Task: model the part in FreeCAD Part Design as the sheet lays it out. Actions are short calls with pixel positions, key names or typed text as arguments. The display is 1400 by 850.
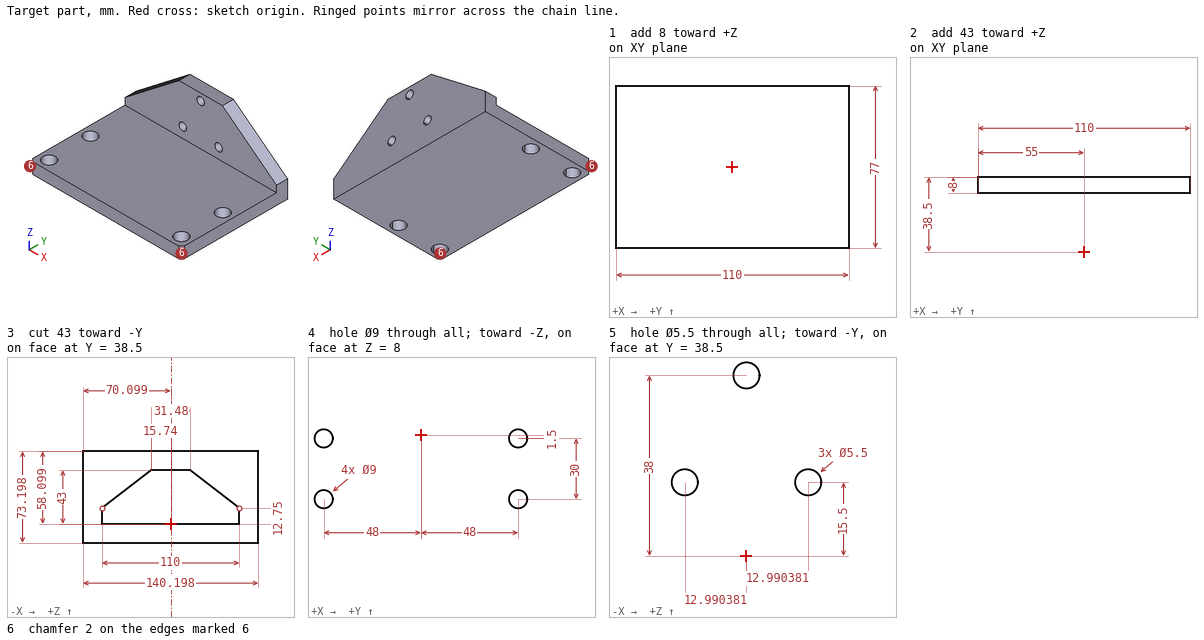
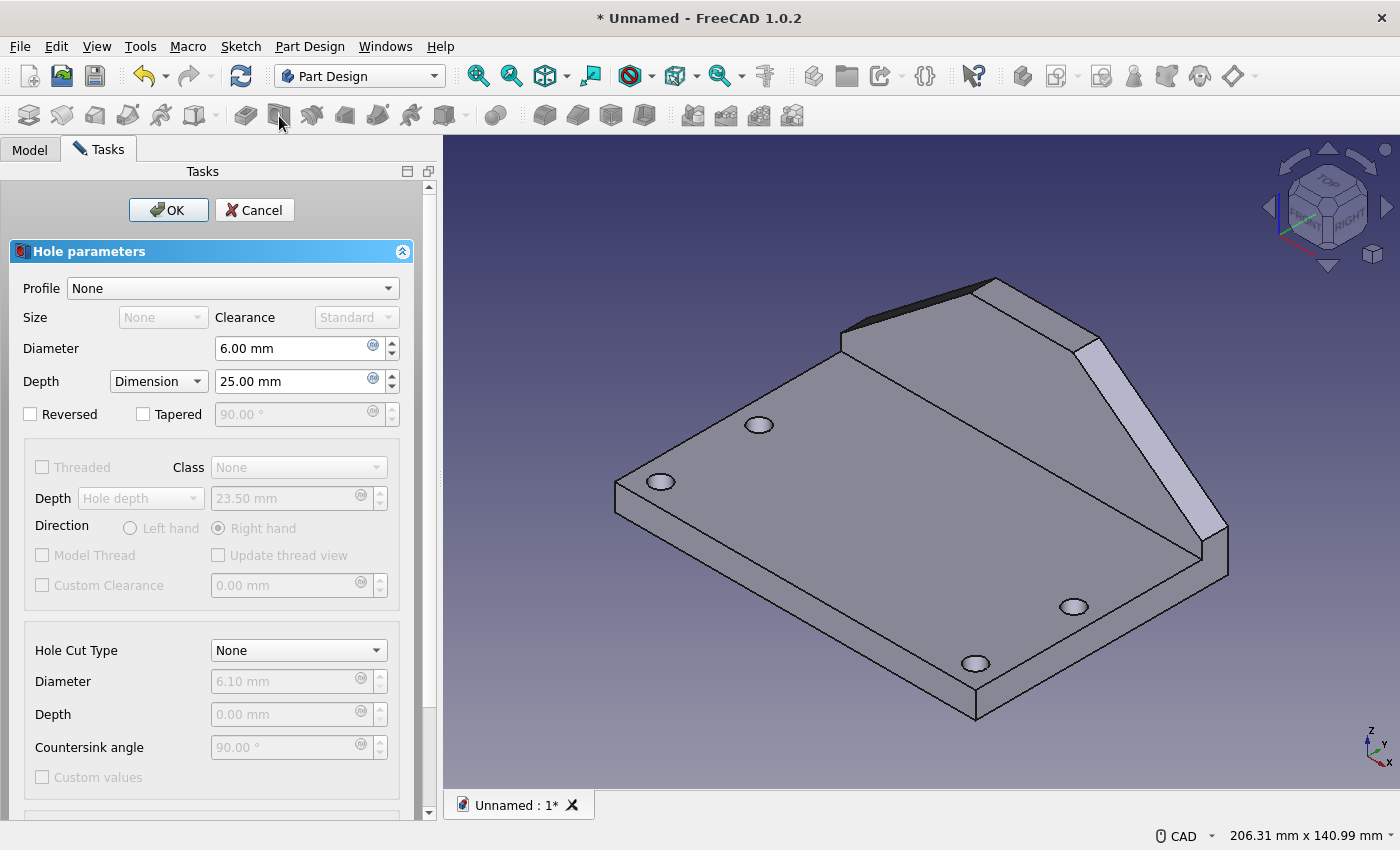
triple_click(300, 348)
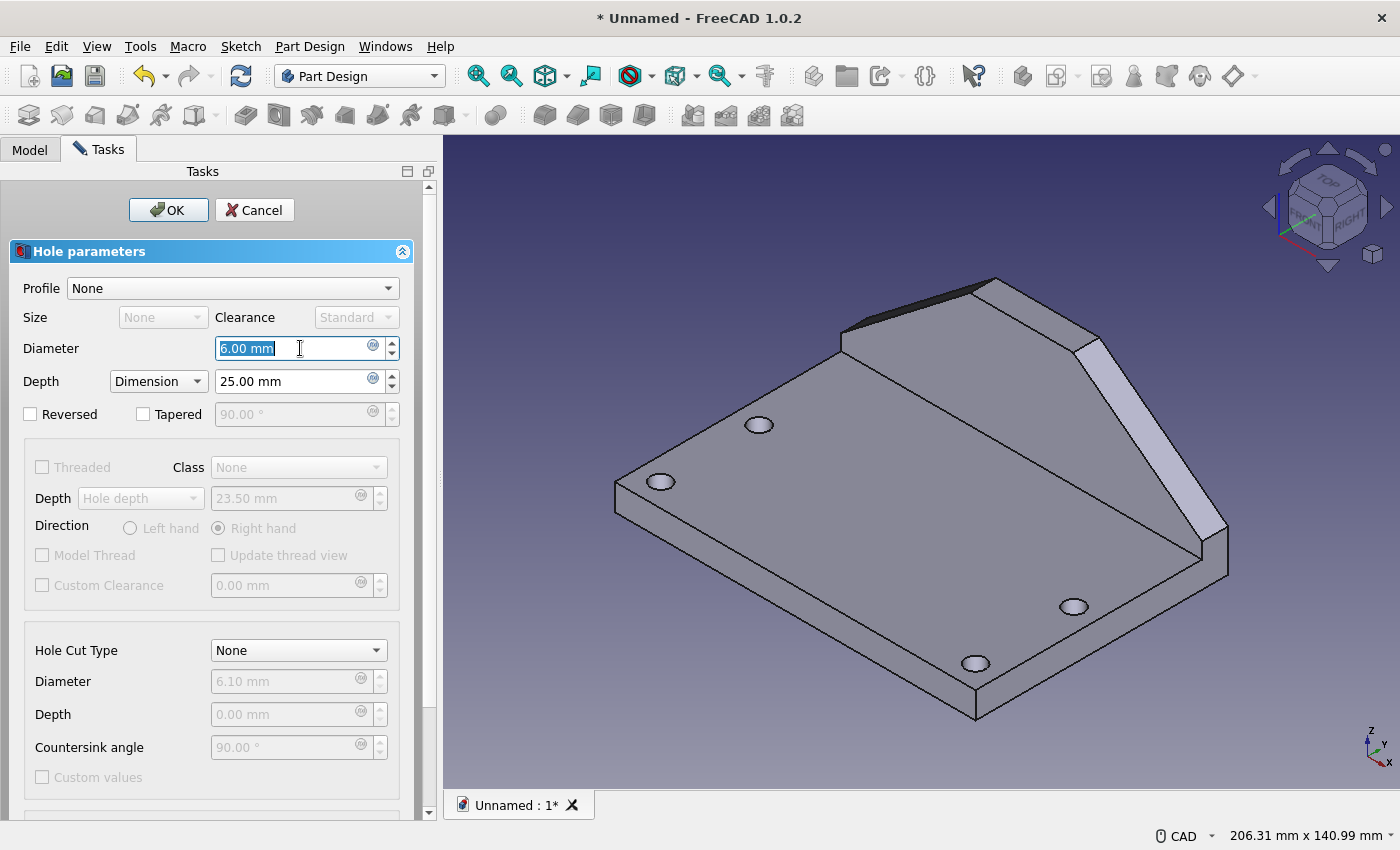
text(9)
key(Tab)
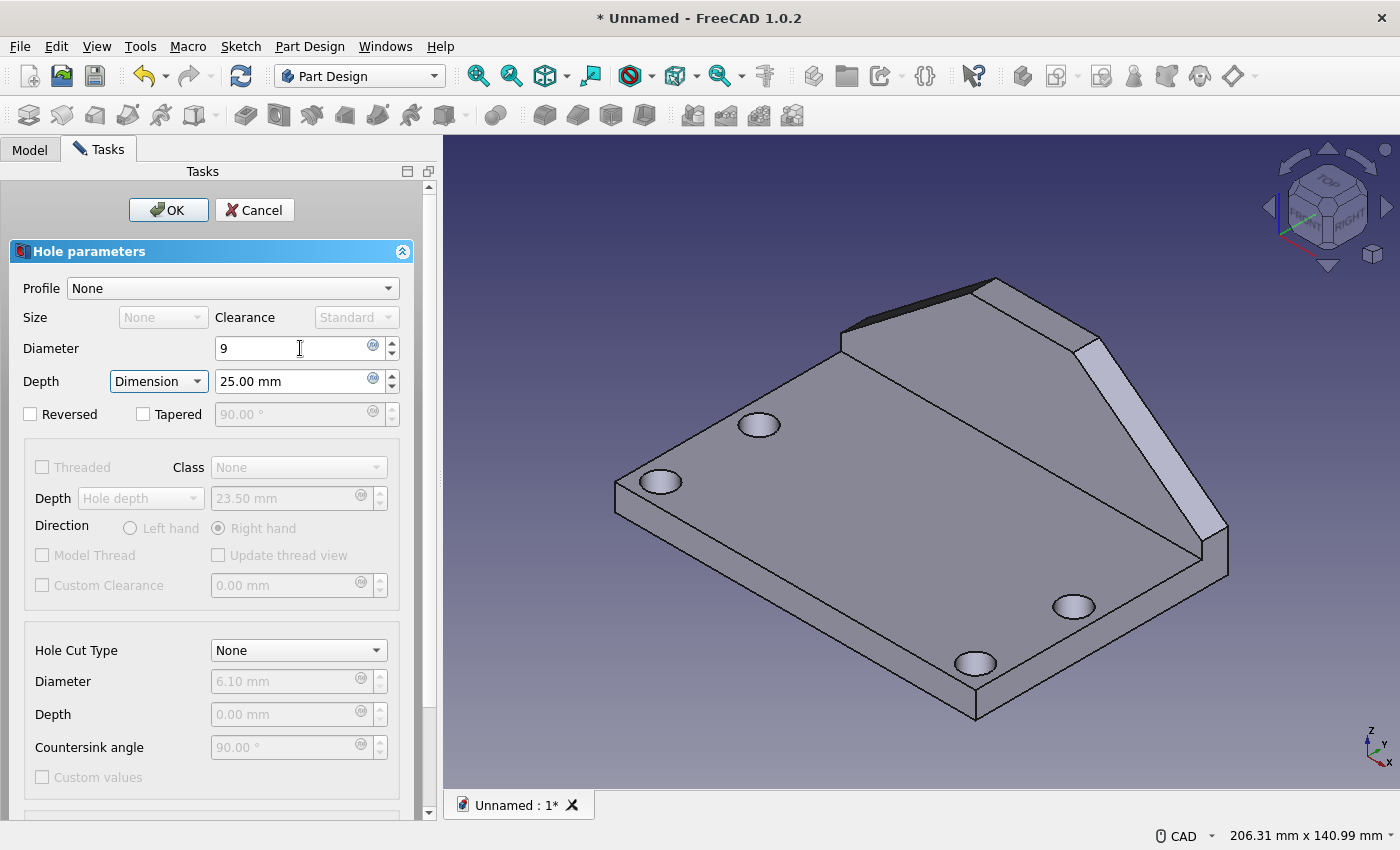
click(160, 382)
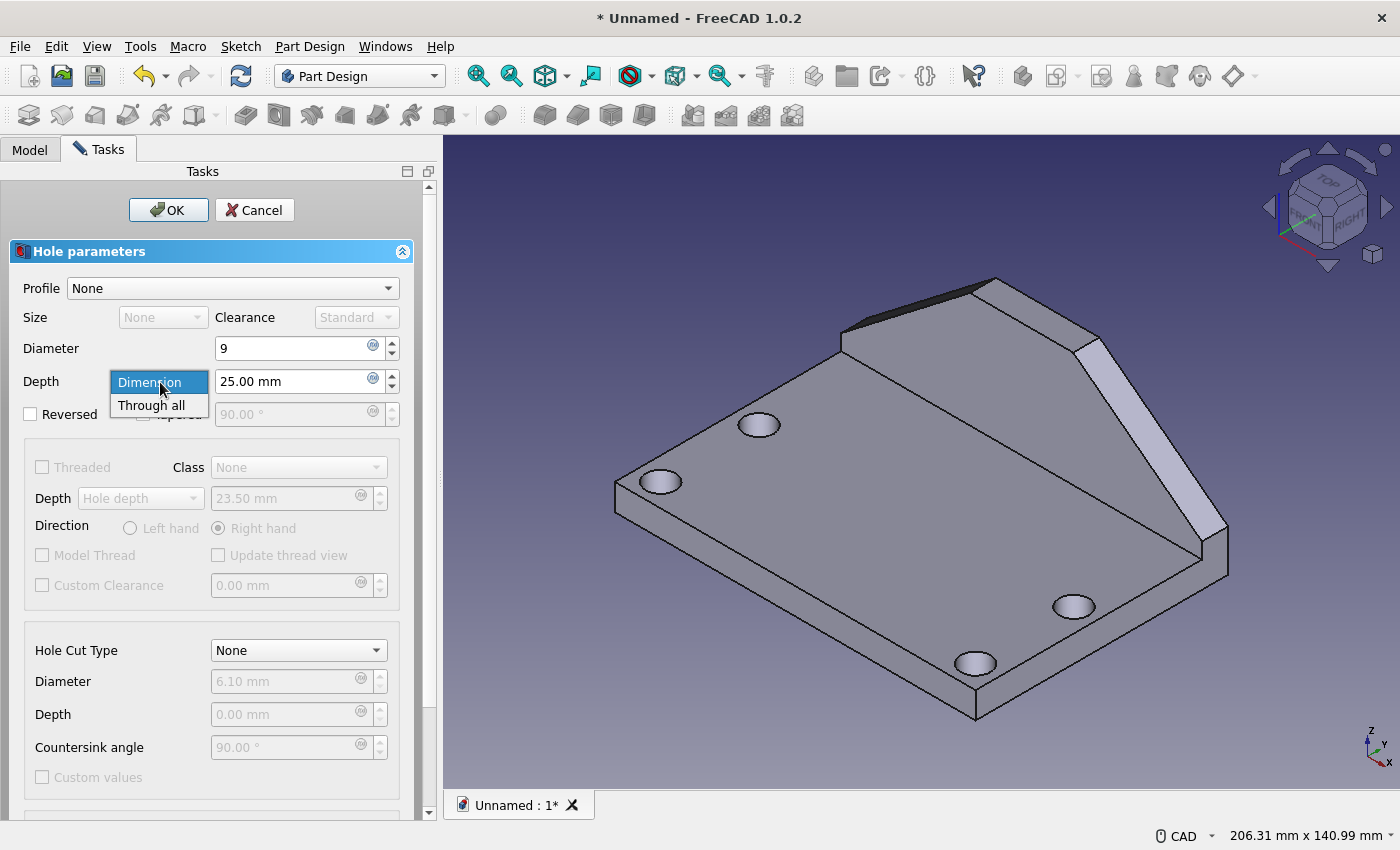
click(158, 406)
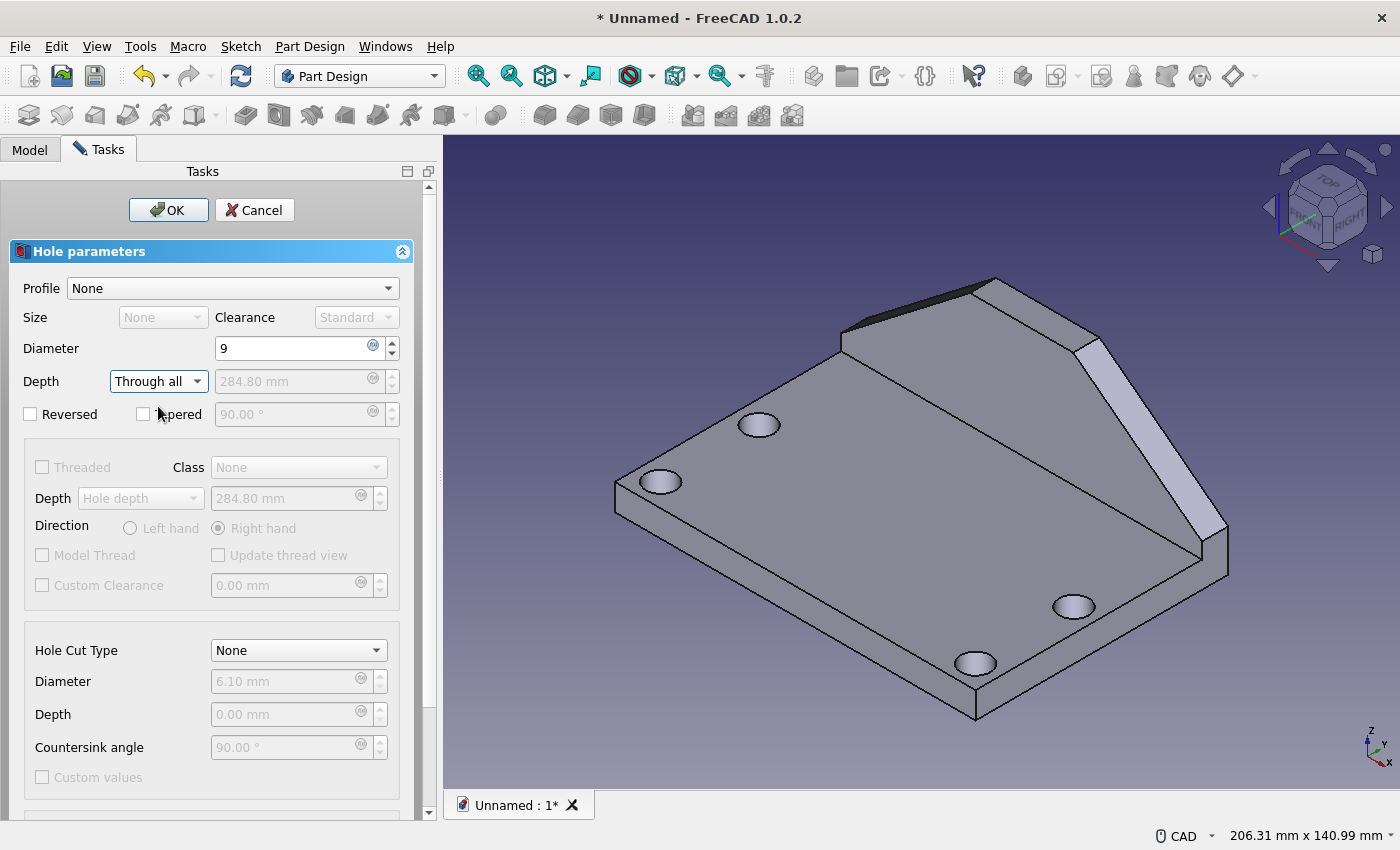
click(169, 210)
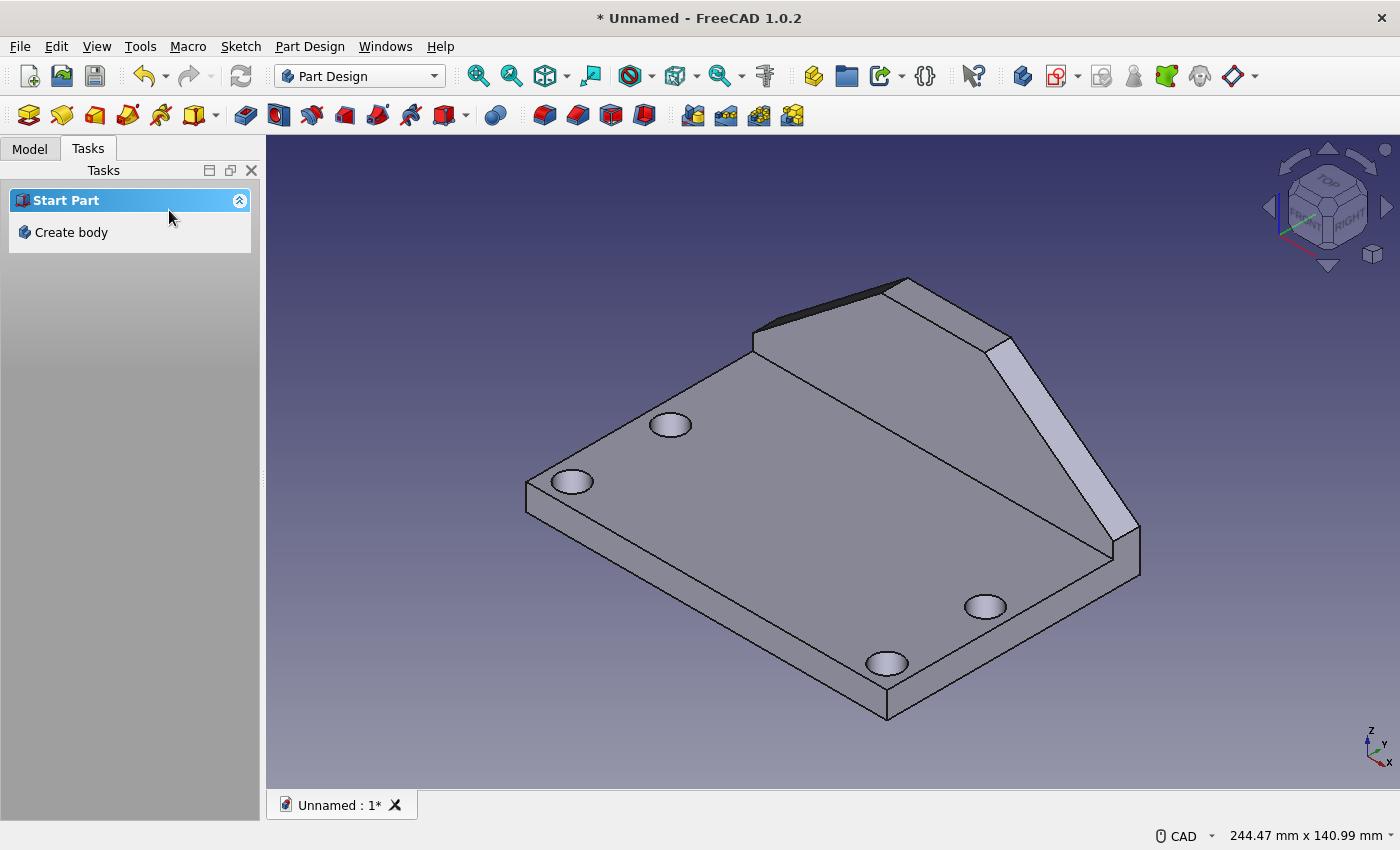
key(4)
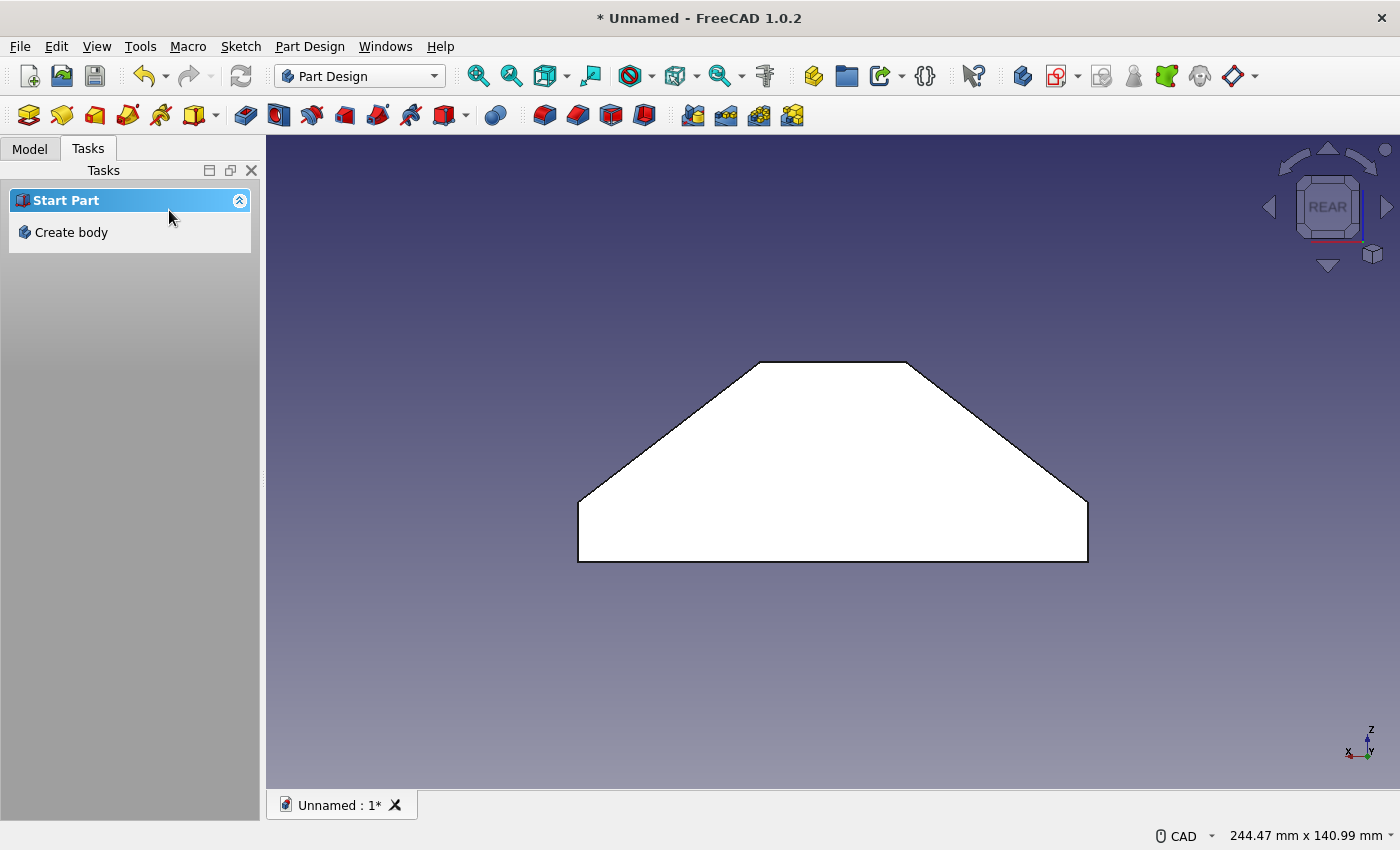
key(v)
key(f)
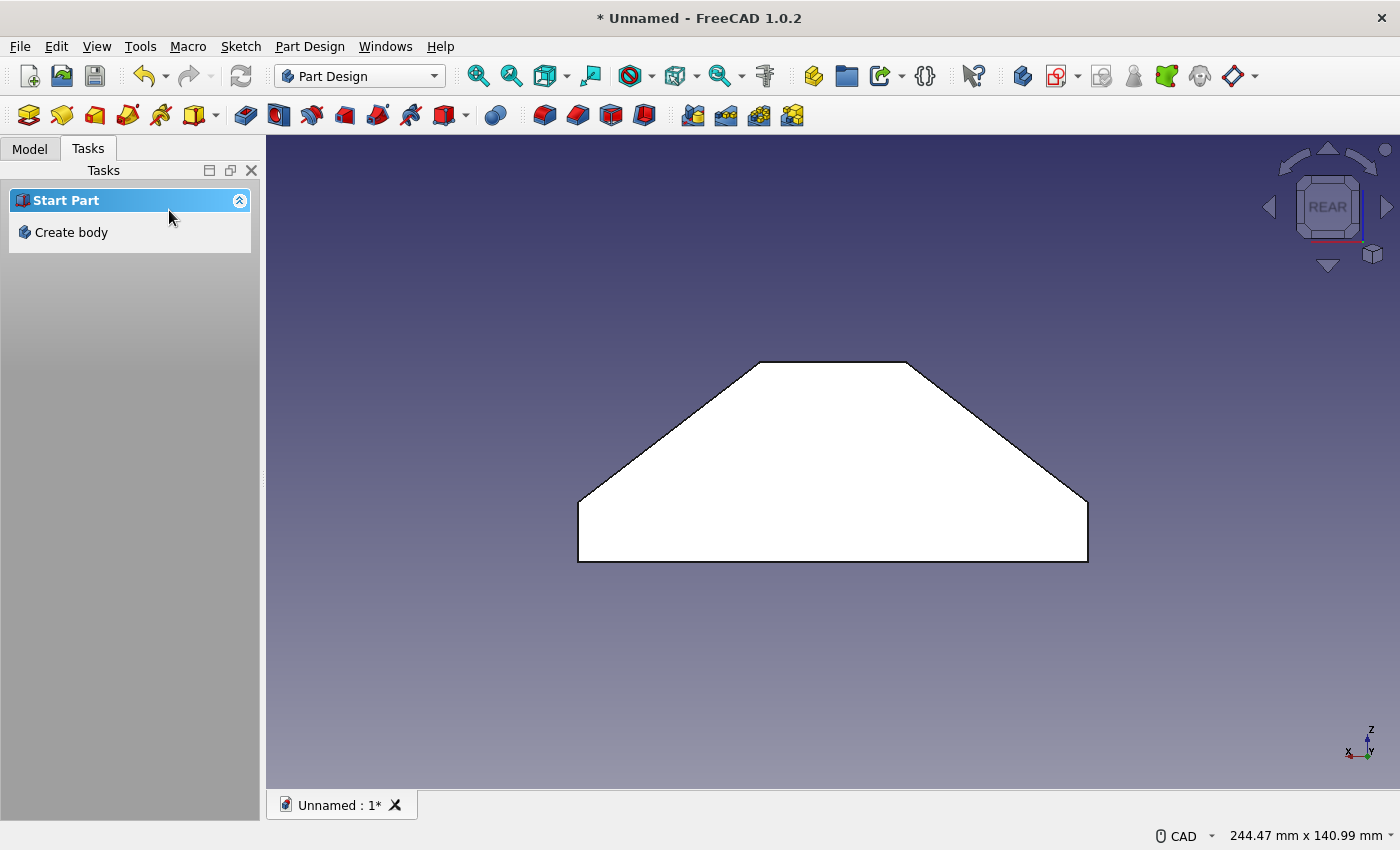
click(833, 461)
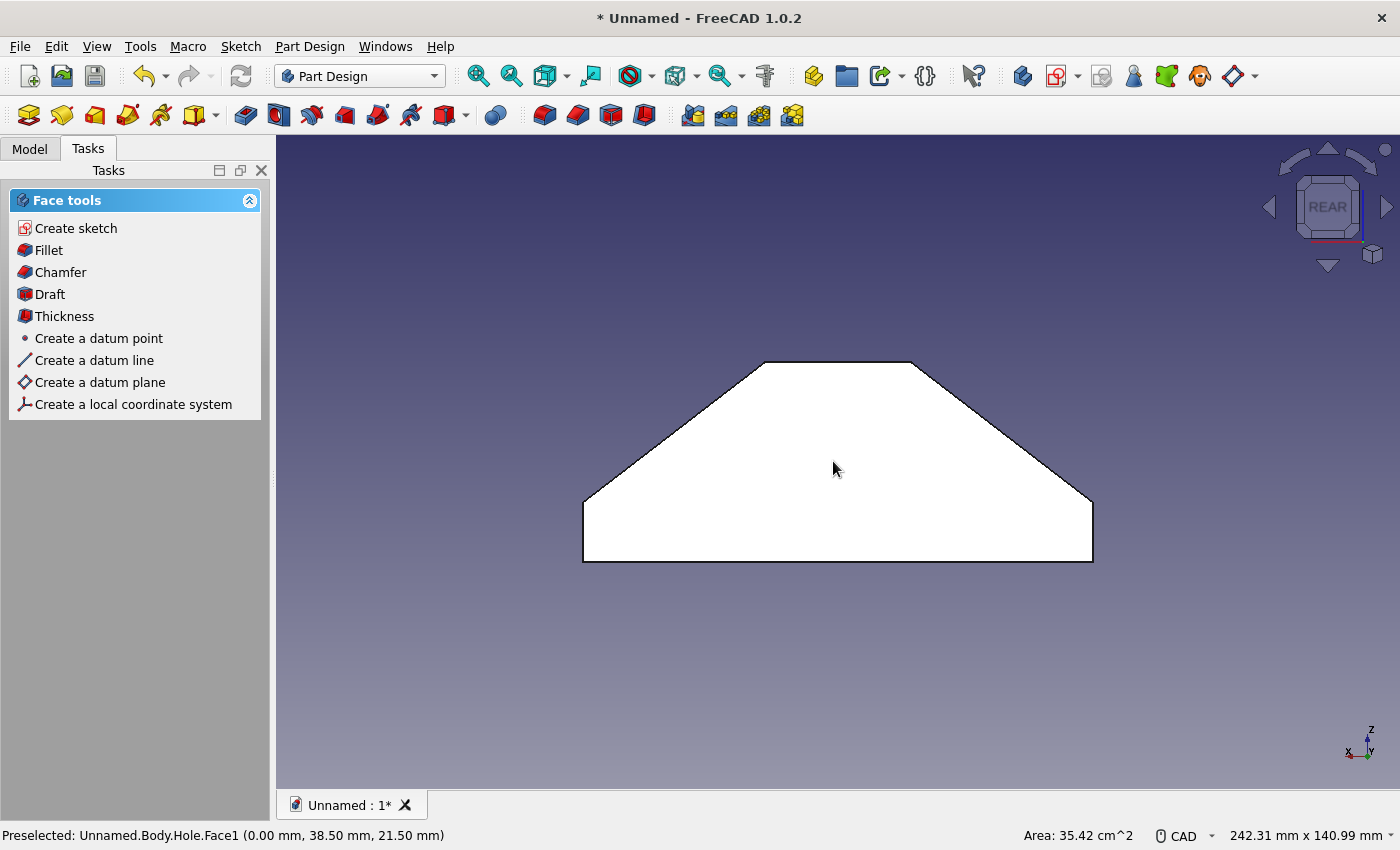
click(1056, 76)